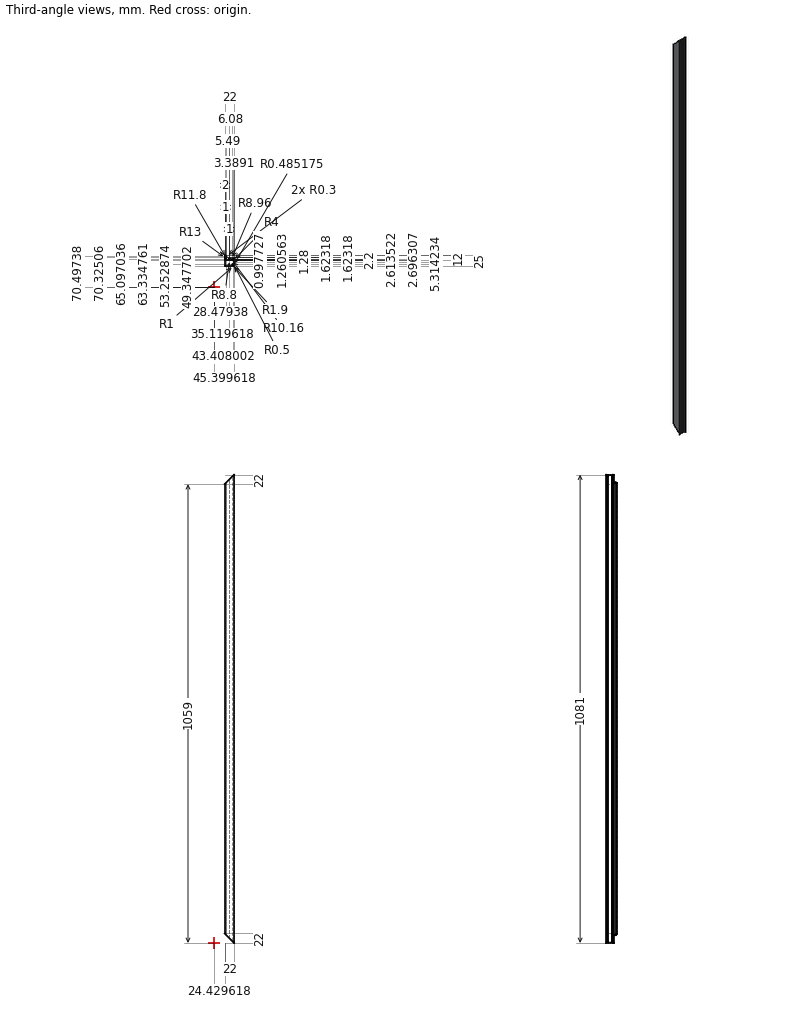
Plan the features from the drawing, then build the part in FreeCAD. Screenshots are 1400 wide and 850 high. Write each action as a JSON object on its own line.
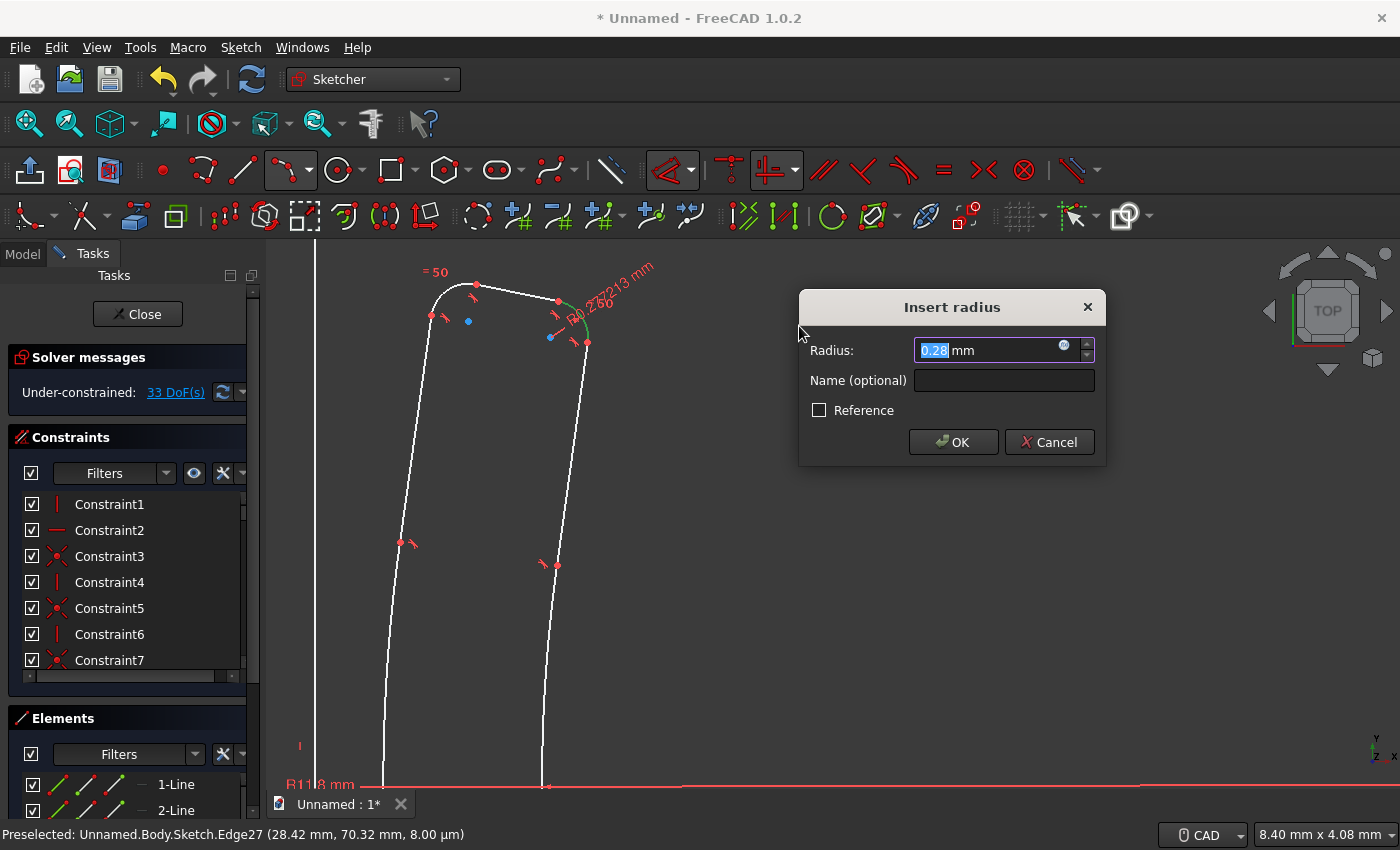
{"action": "type", "text": "0.3"}
{"action": "key", "text": "Return"}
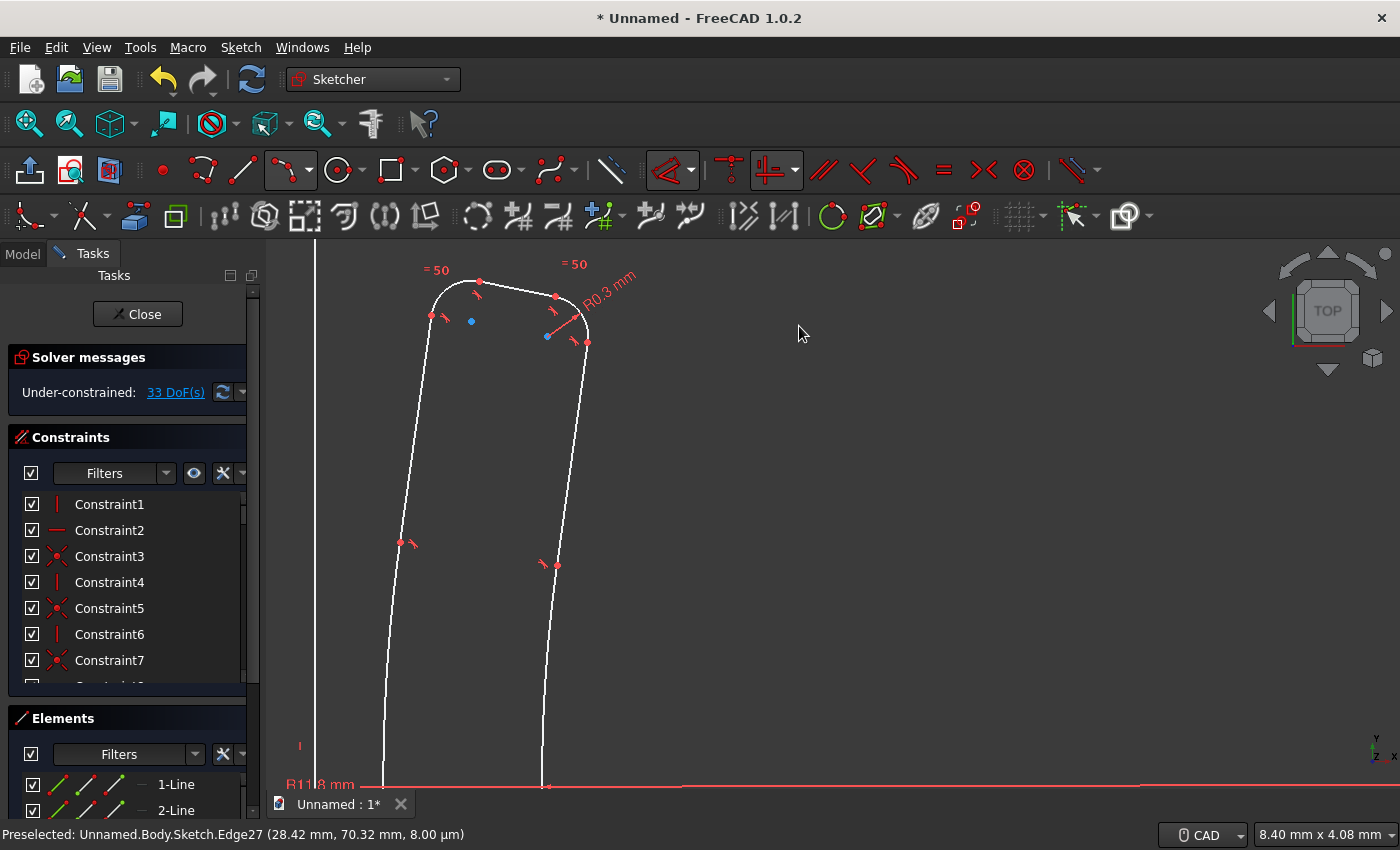
{"action": "scroll", "coordinate": [669, 377], "scroll_direction": "down", "scroll_amount": 11}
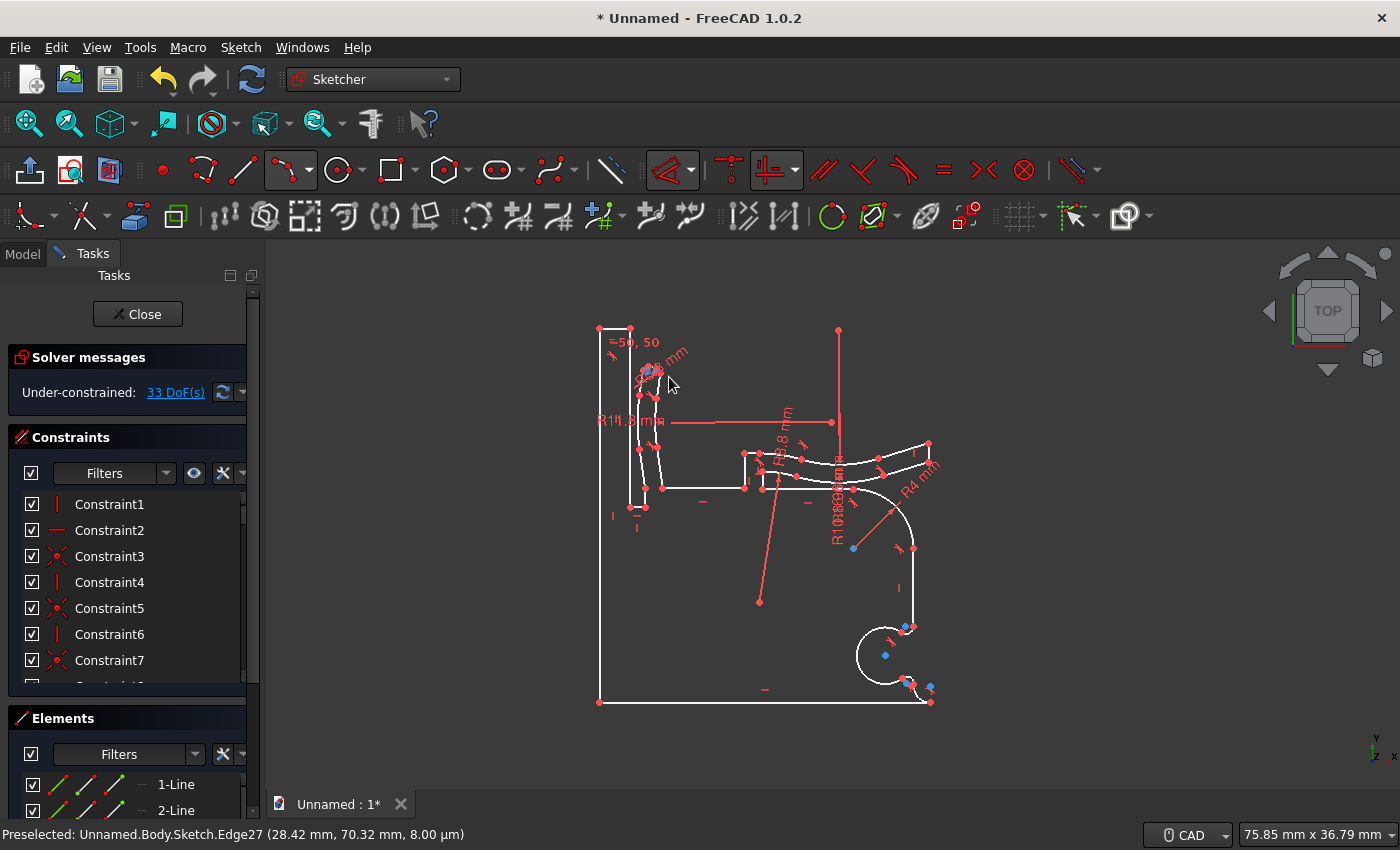
{"action": "scroll", "coordinate": [638, 412], "scroll_direction": "up", "scroll_amount": 3}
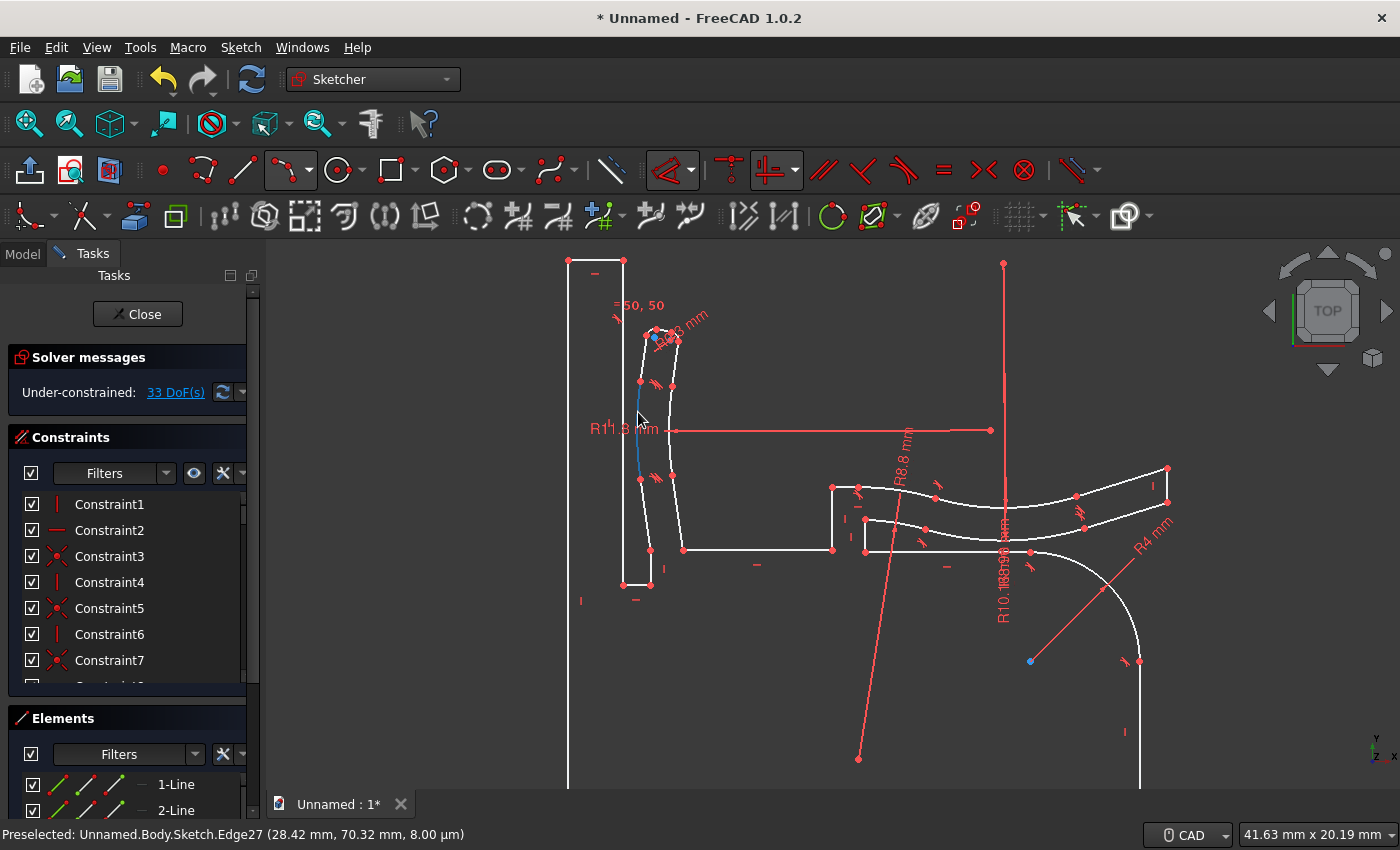
{"action": "left_click", "coordinate": [638, 411]}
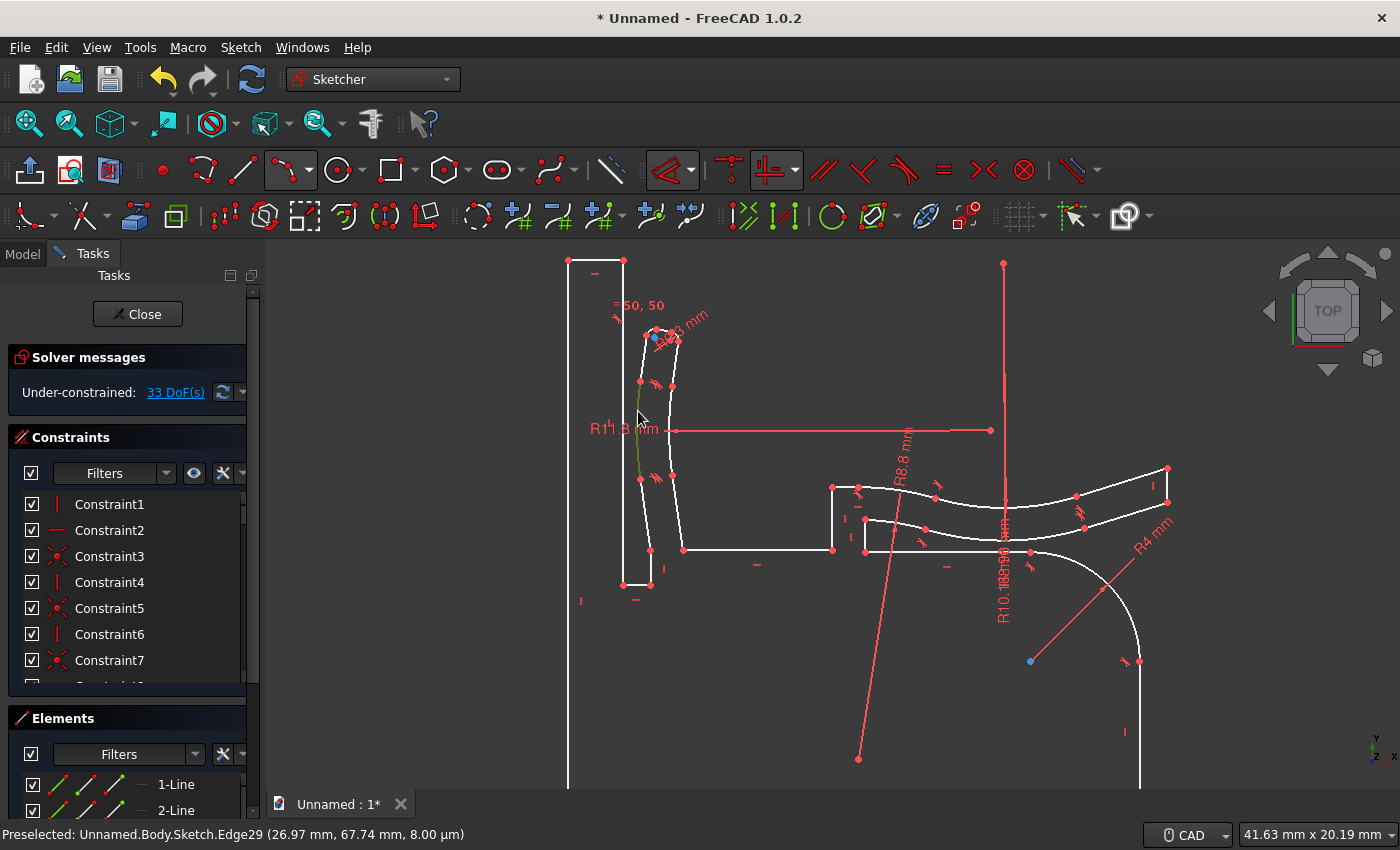
{"action": "left_click", "coordinate": [694, 170]}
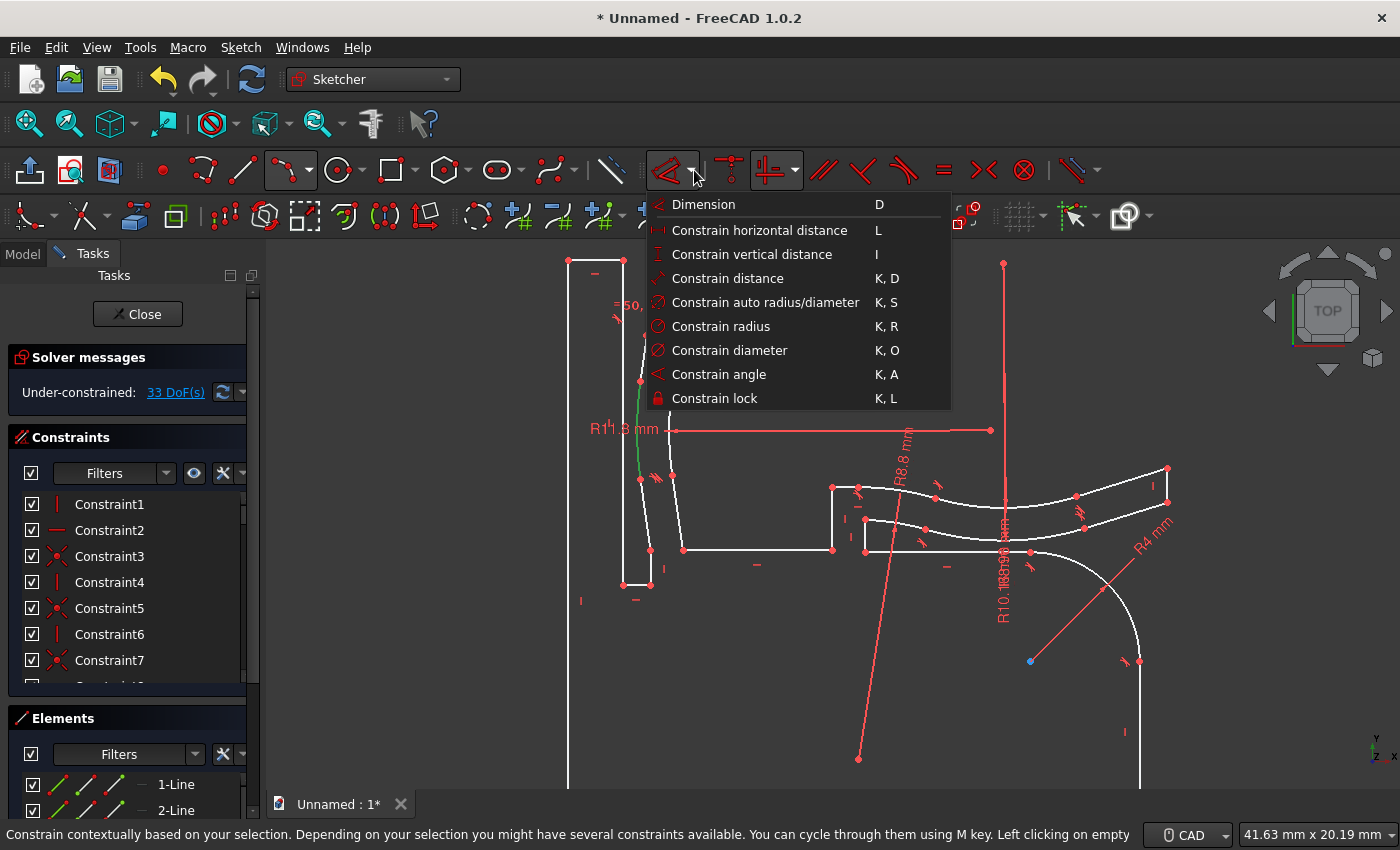
{"action": "left_click", "coordinate": [799, 326]}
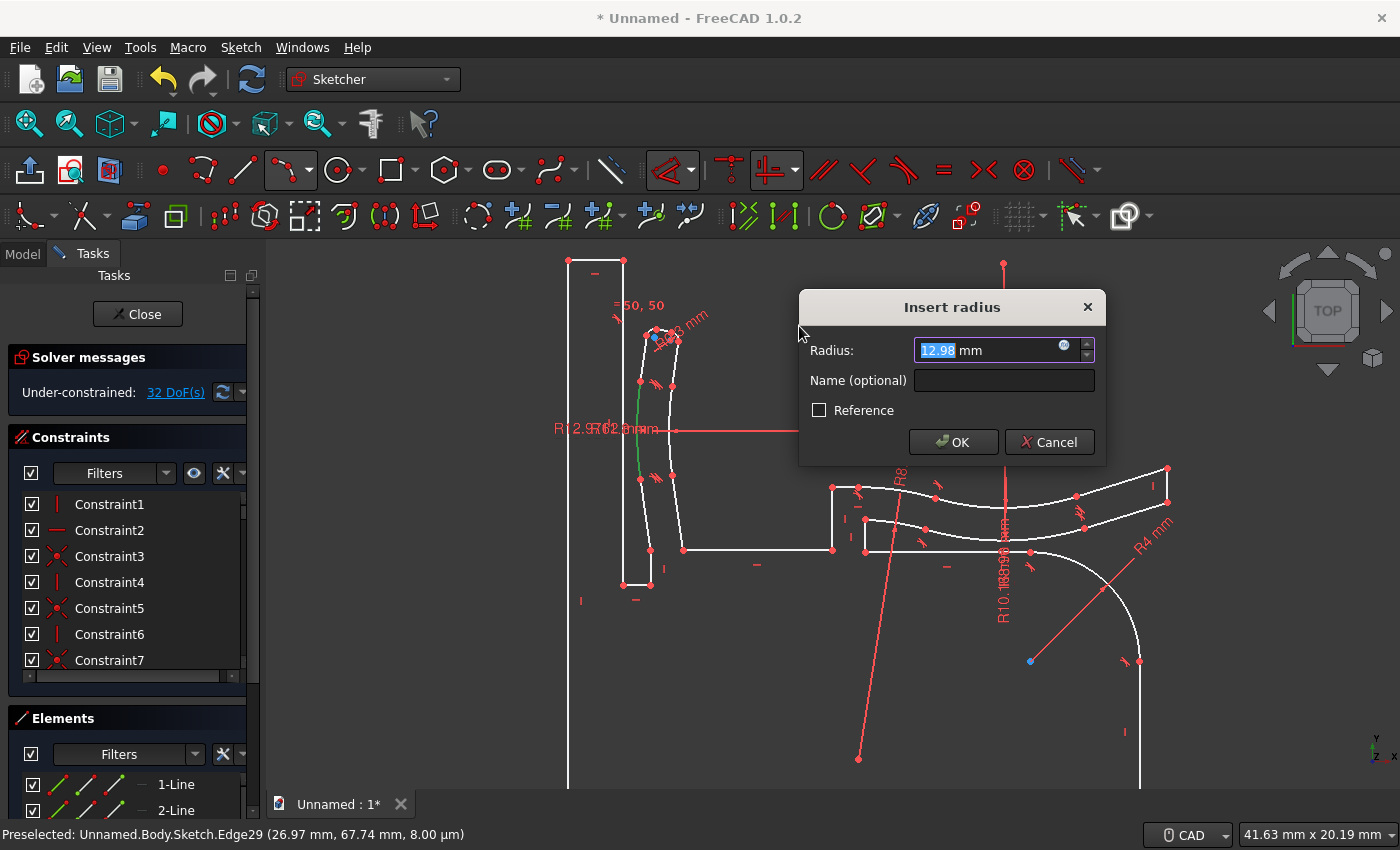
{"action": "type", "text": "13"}
{"action": "key", "text": "Return"}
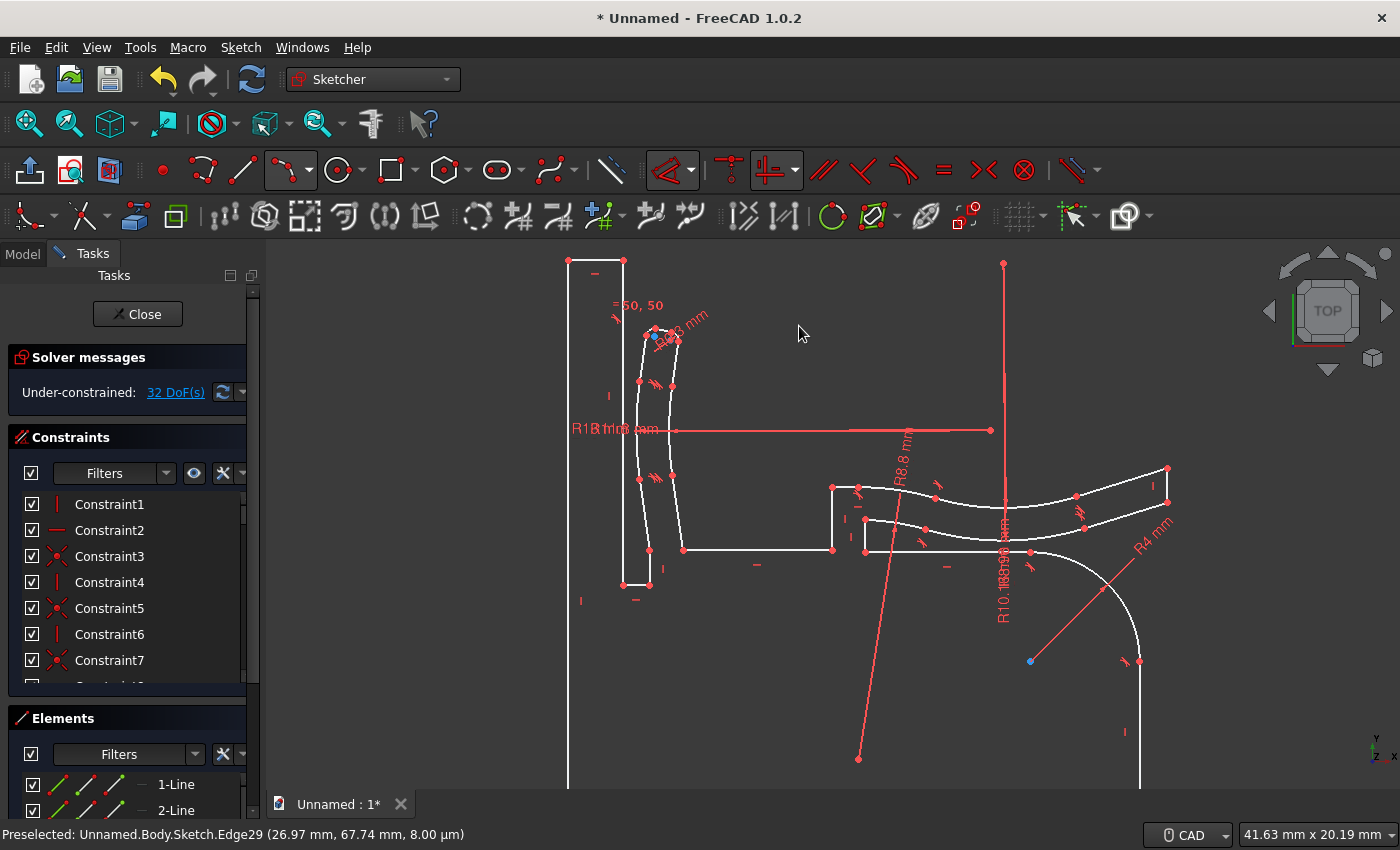
{"action": "scroll", "coordinate": [638, 411], "scroll_direction": "down", "scroll_amount": 3}